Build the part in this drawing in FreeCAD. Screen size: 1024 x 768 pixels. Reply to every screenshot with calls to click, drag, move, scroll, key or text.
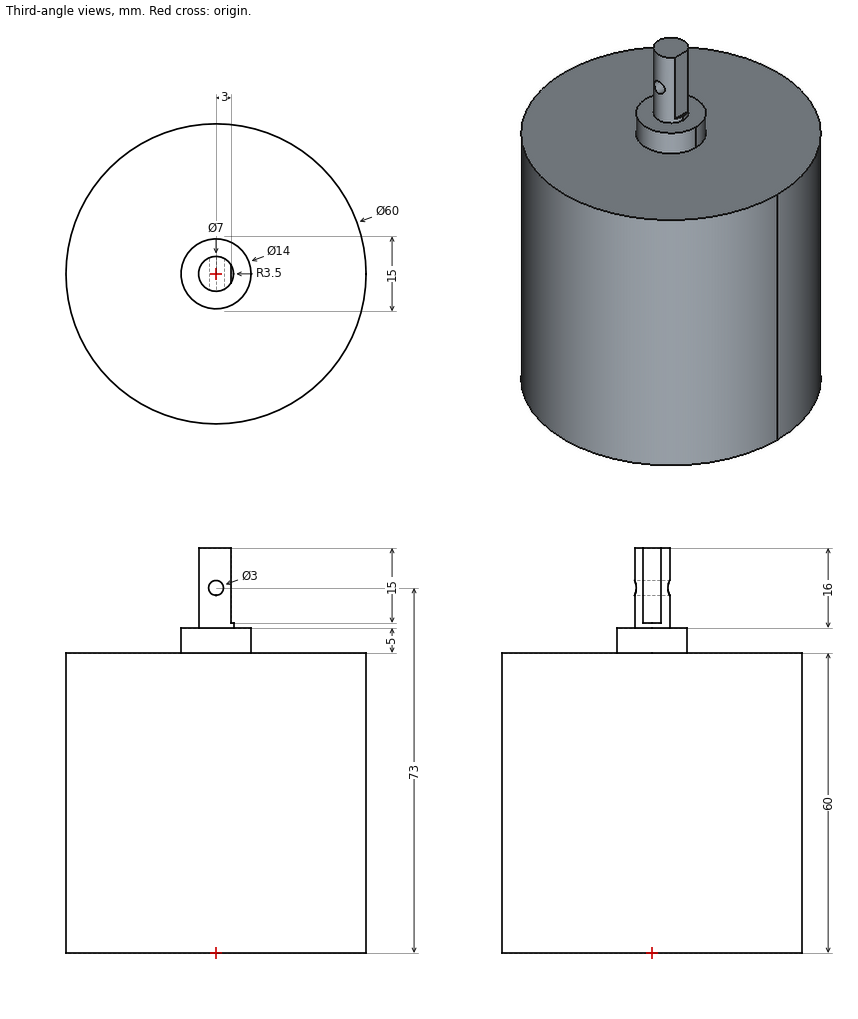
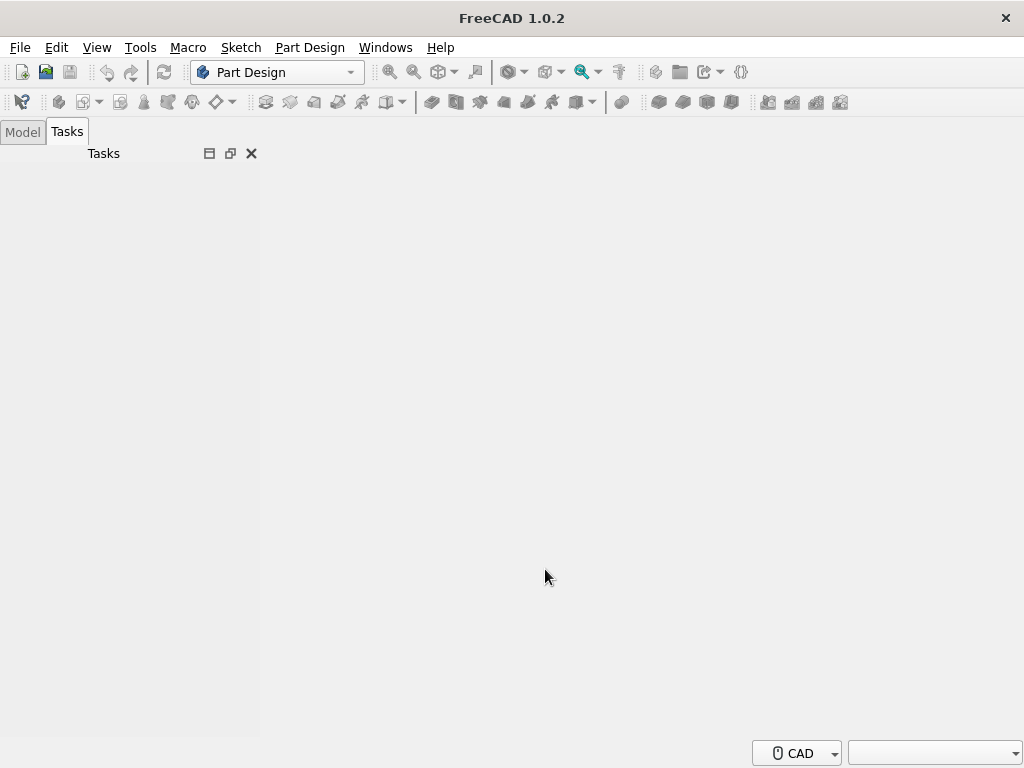
click(22, 72)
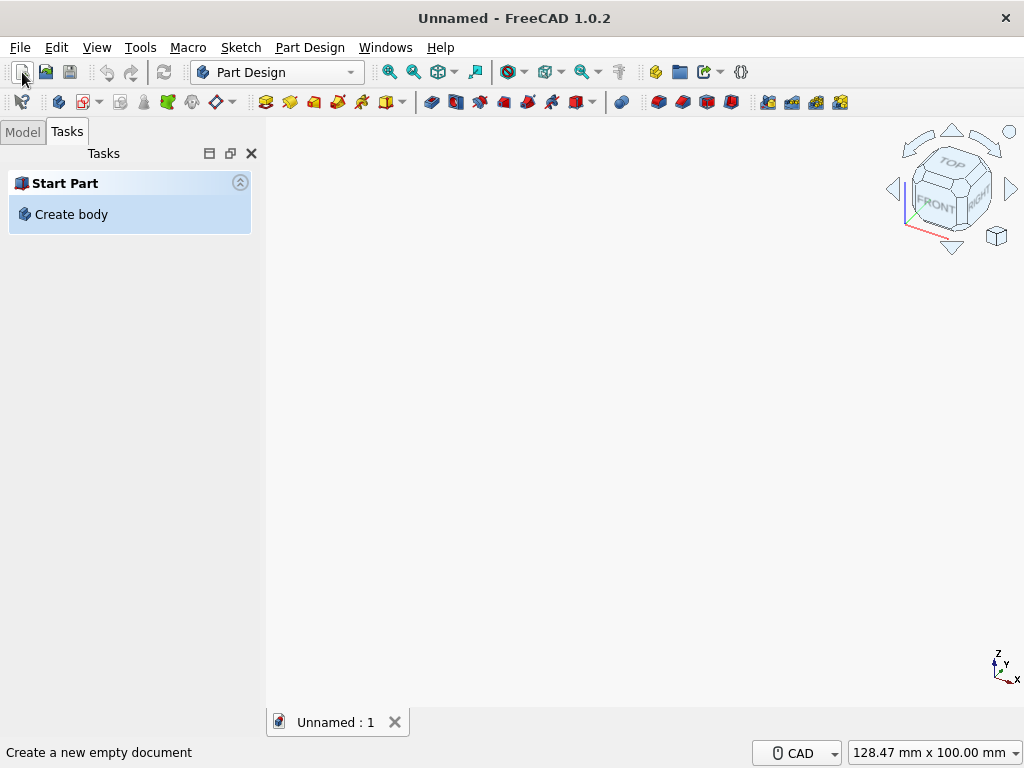
click(84, 102)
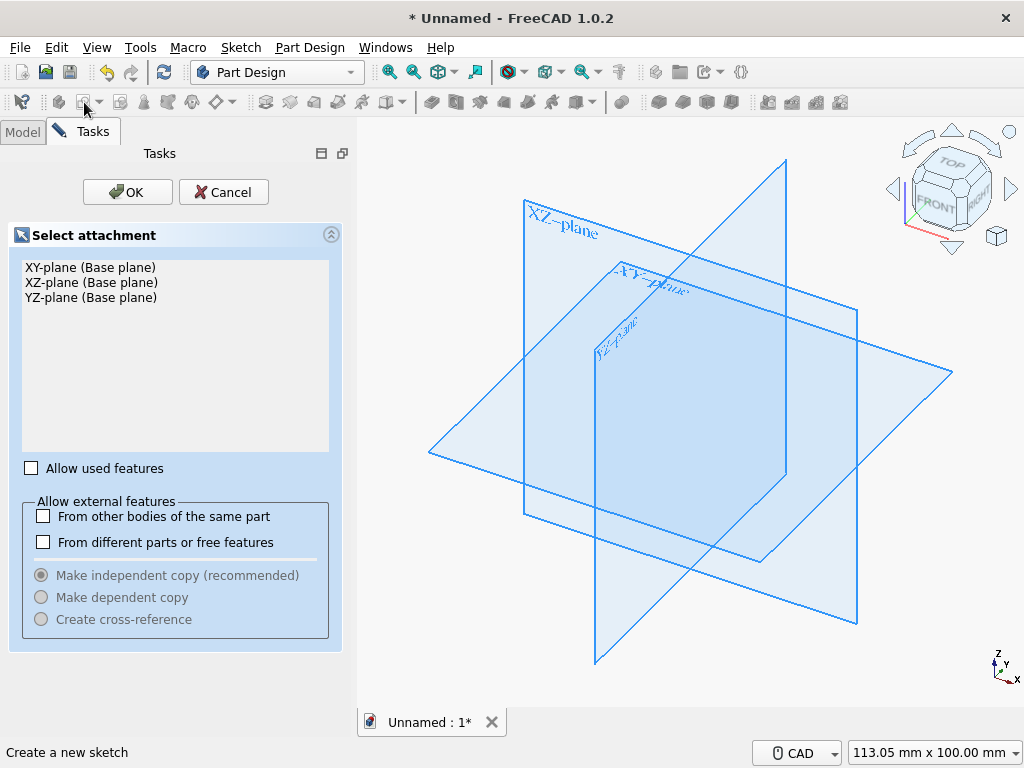
click(82, 268)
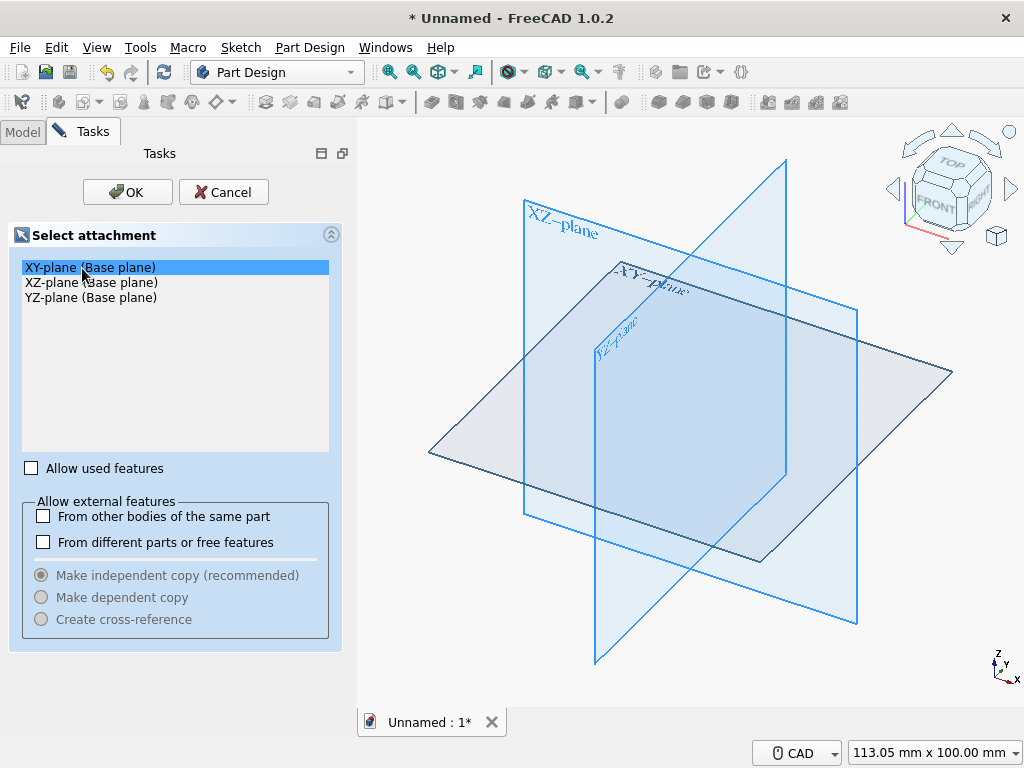
click(128, 192)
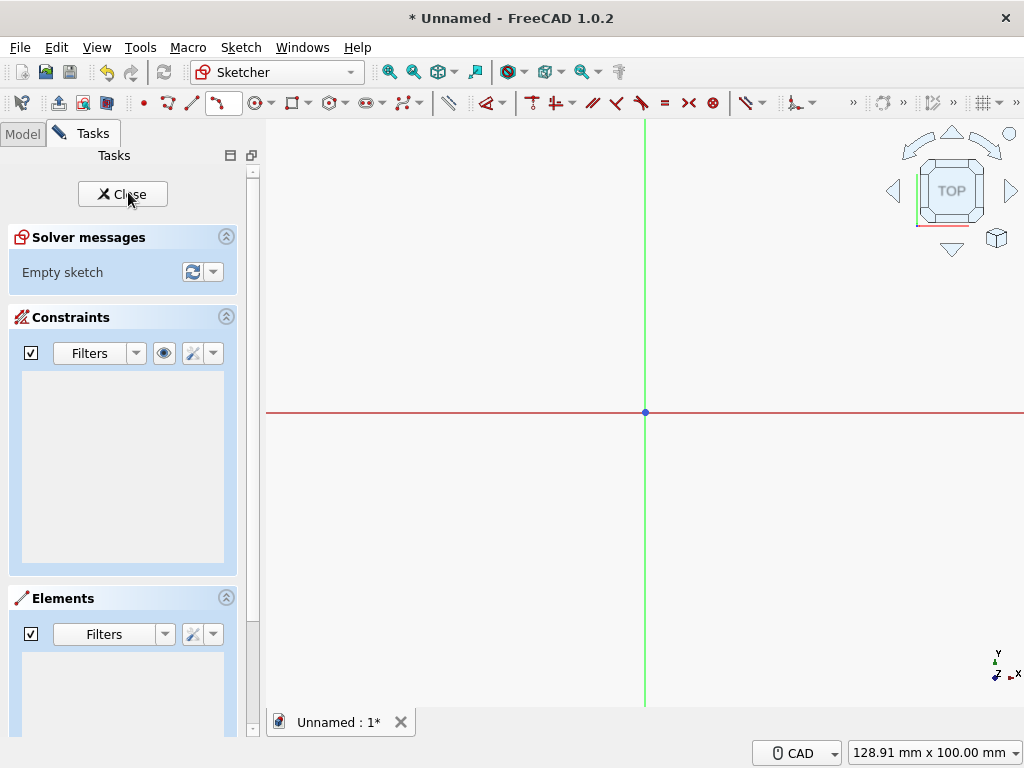
click(256, 104)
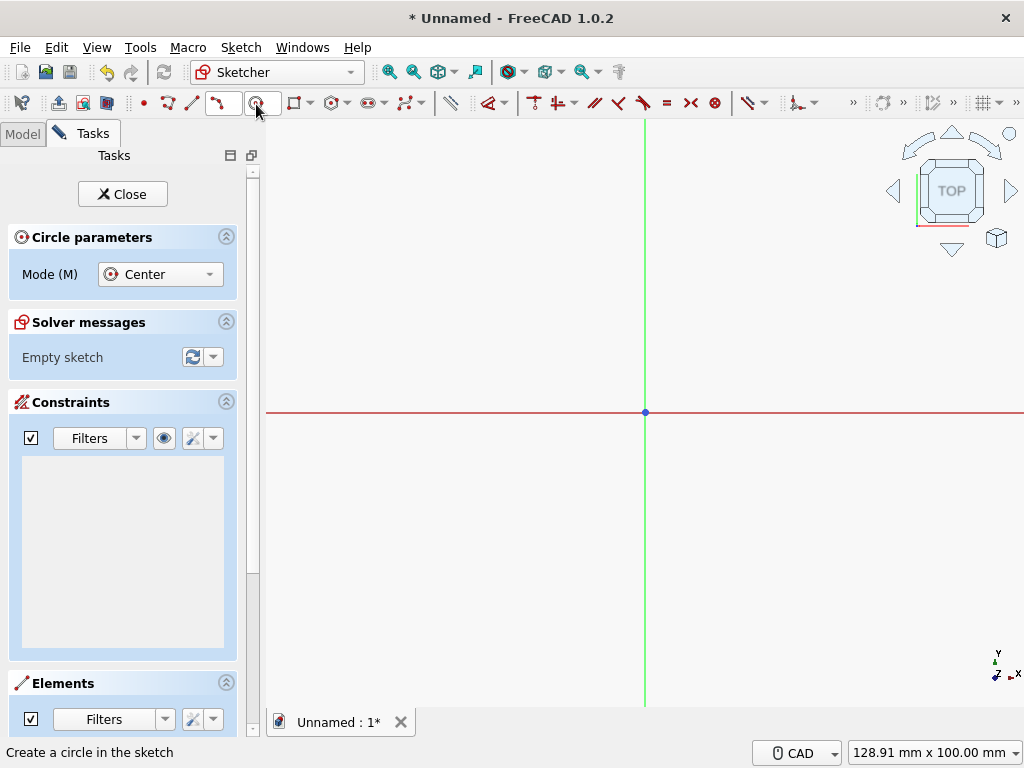
click(645, 413)
move(770, 288)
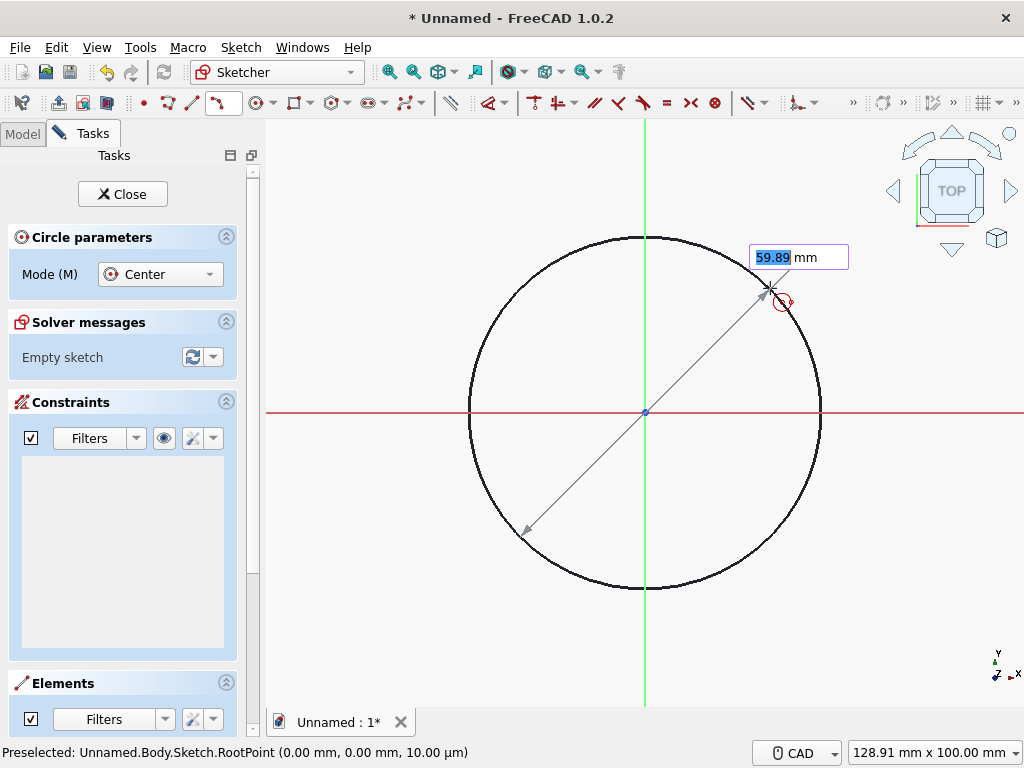
text(60)
key(Return)
key(Escape)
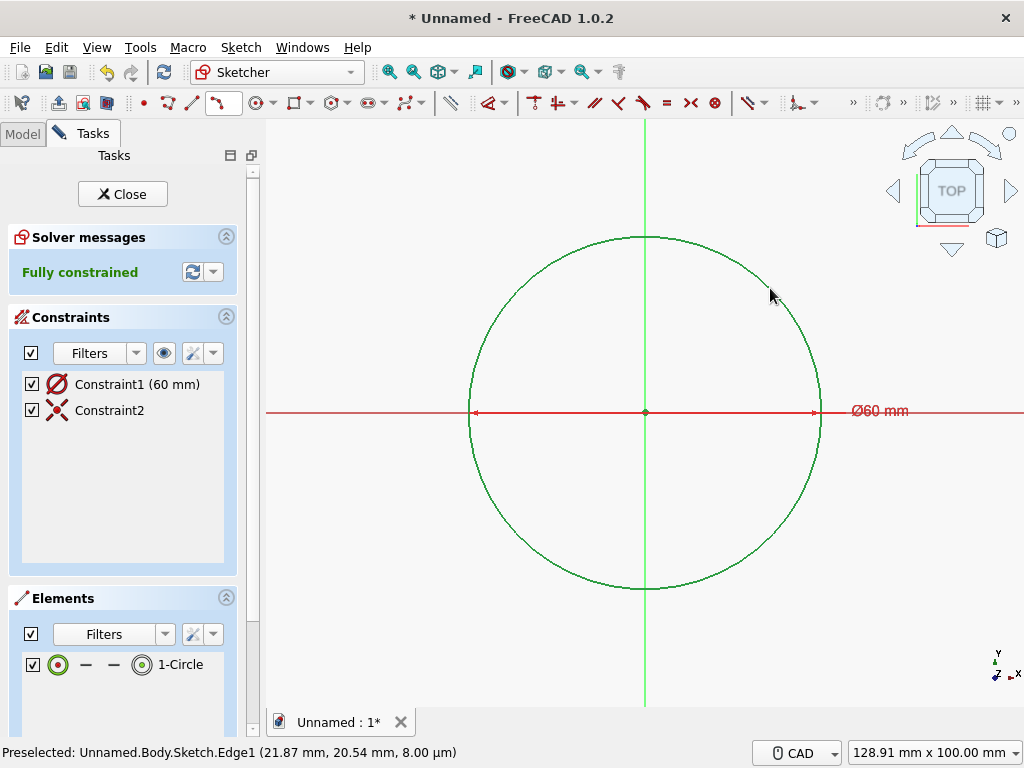
click(123, 194)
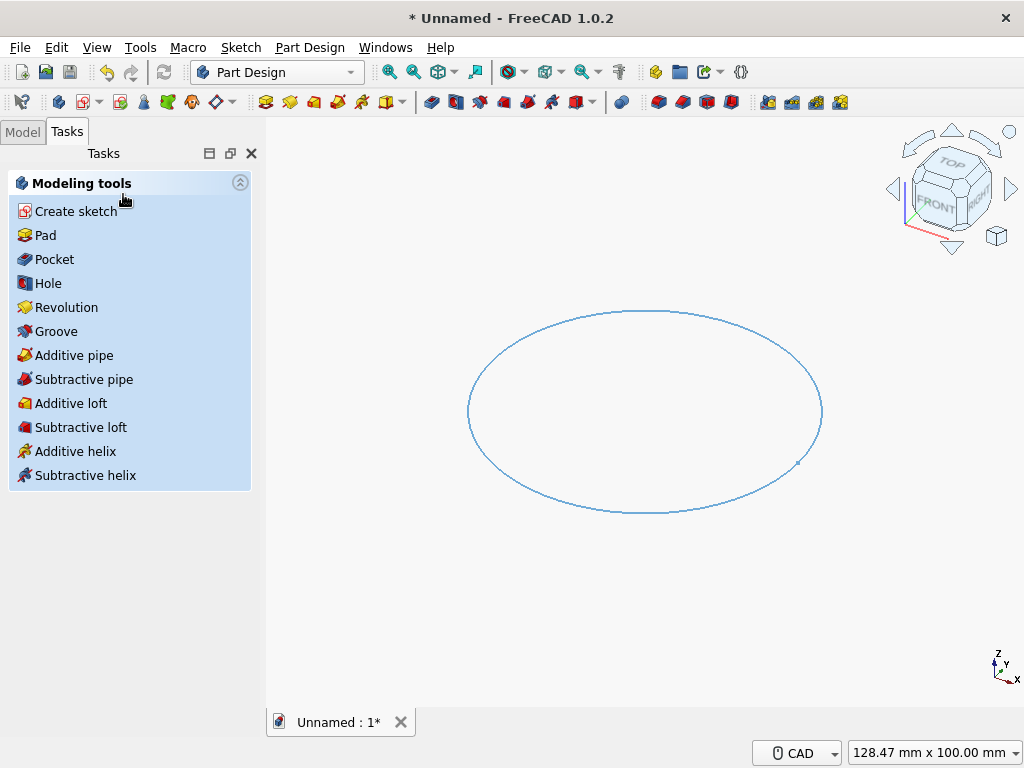
click(266, 102)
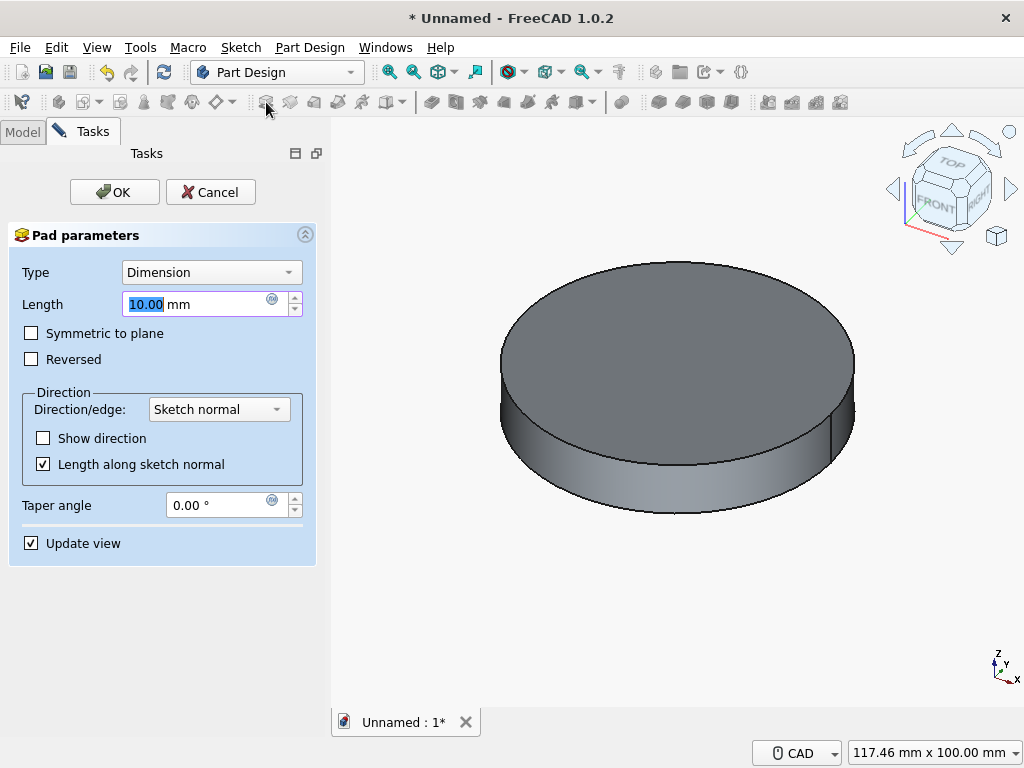
text(60)
key(Tab)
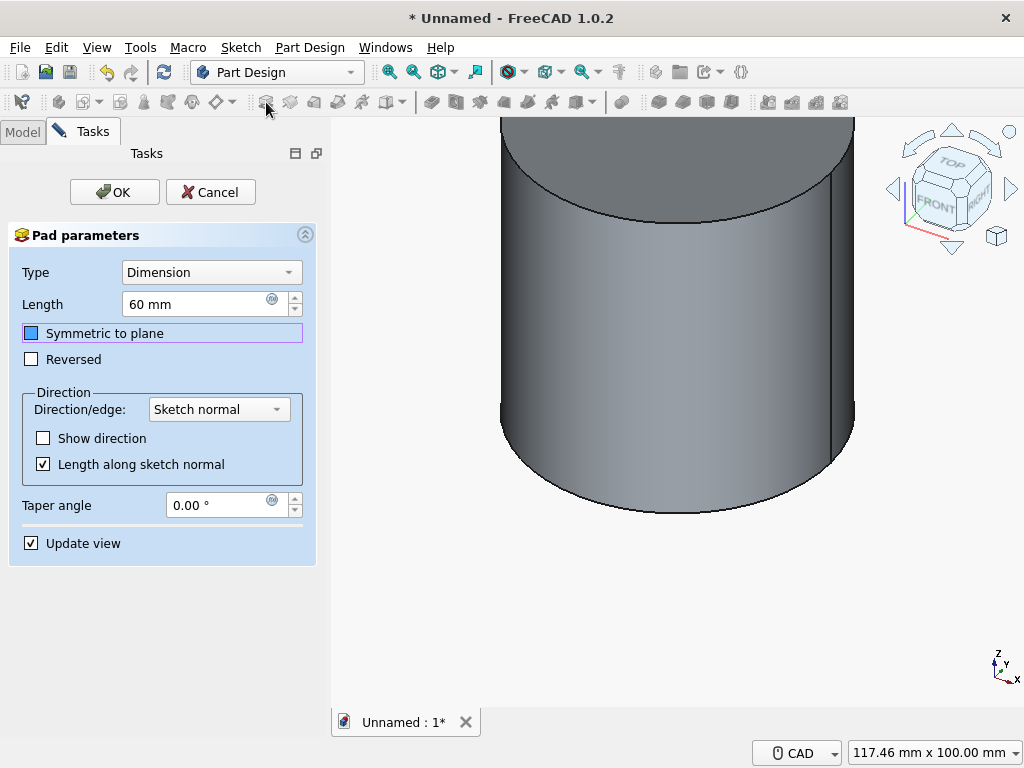
click(115, 192)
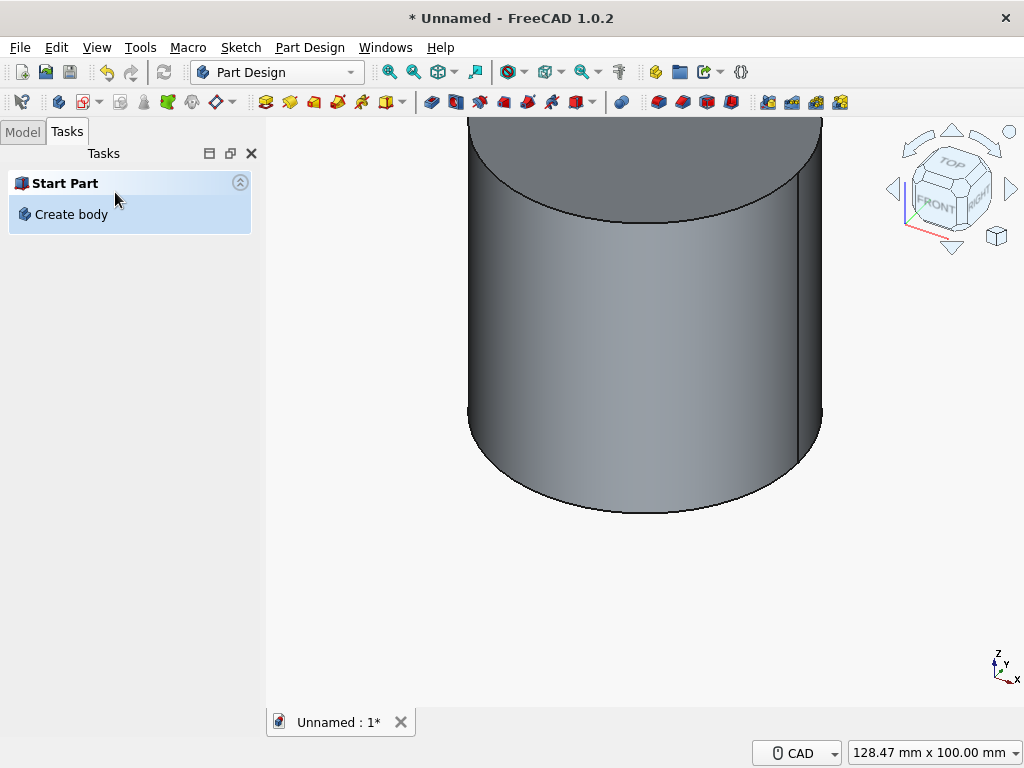
click(390, 72)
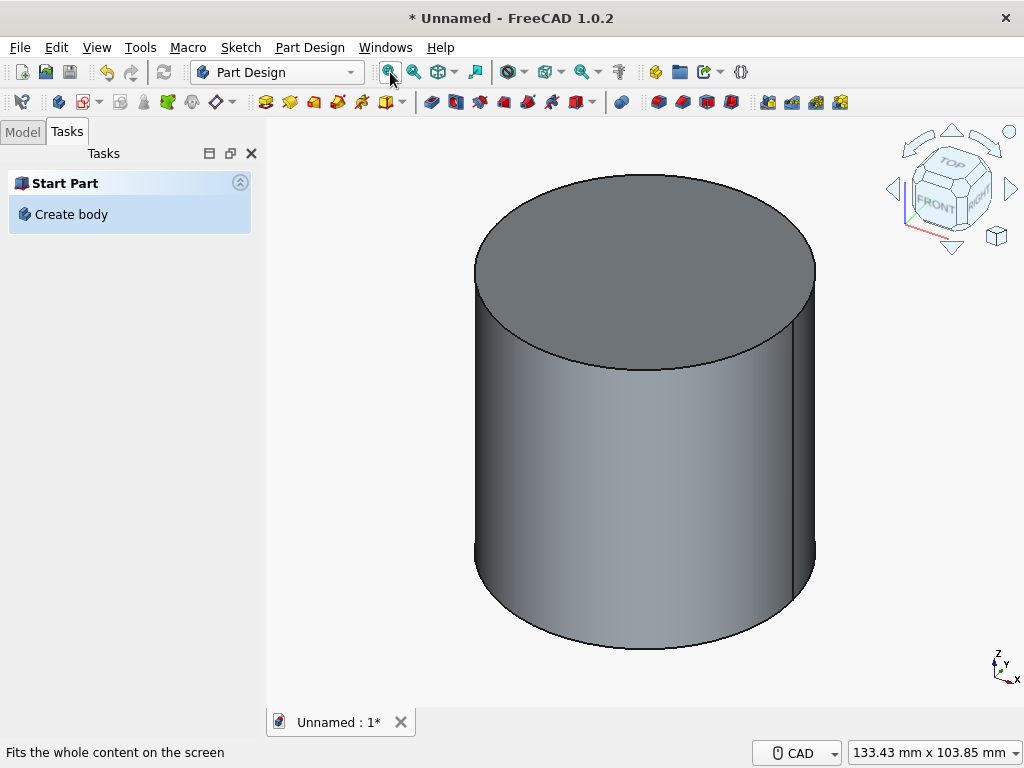
click(645, 271)